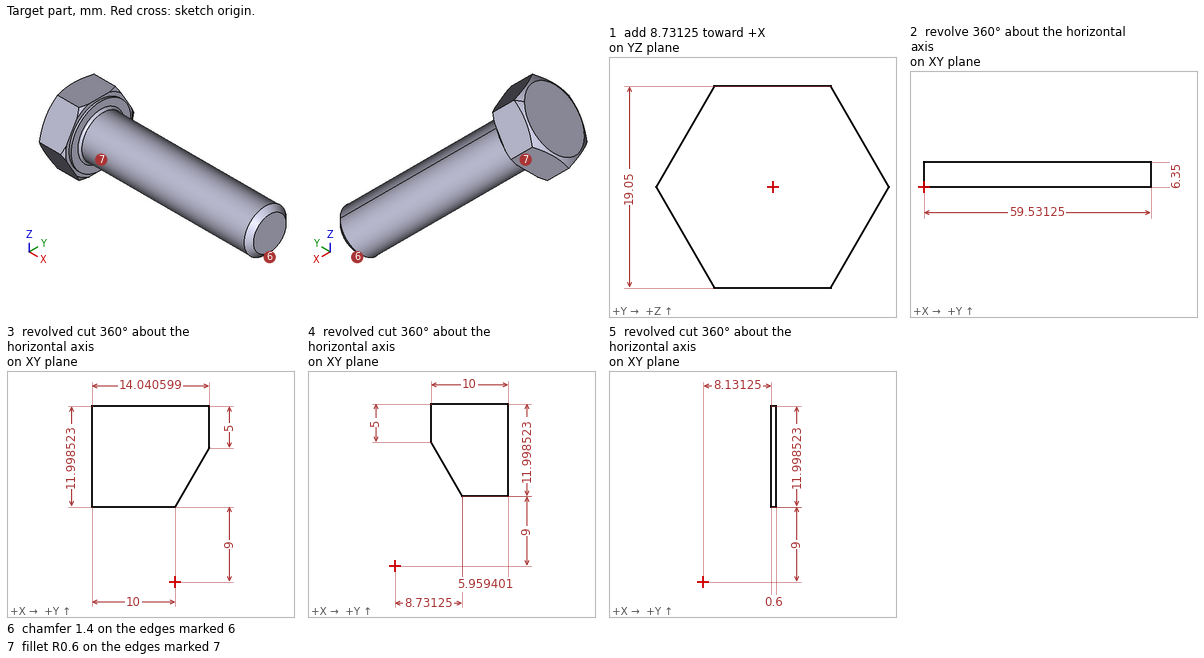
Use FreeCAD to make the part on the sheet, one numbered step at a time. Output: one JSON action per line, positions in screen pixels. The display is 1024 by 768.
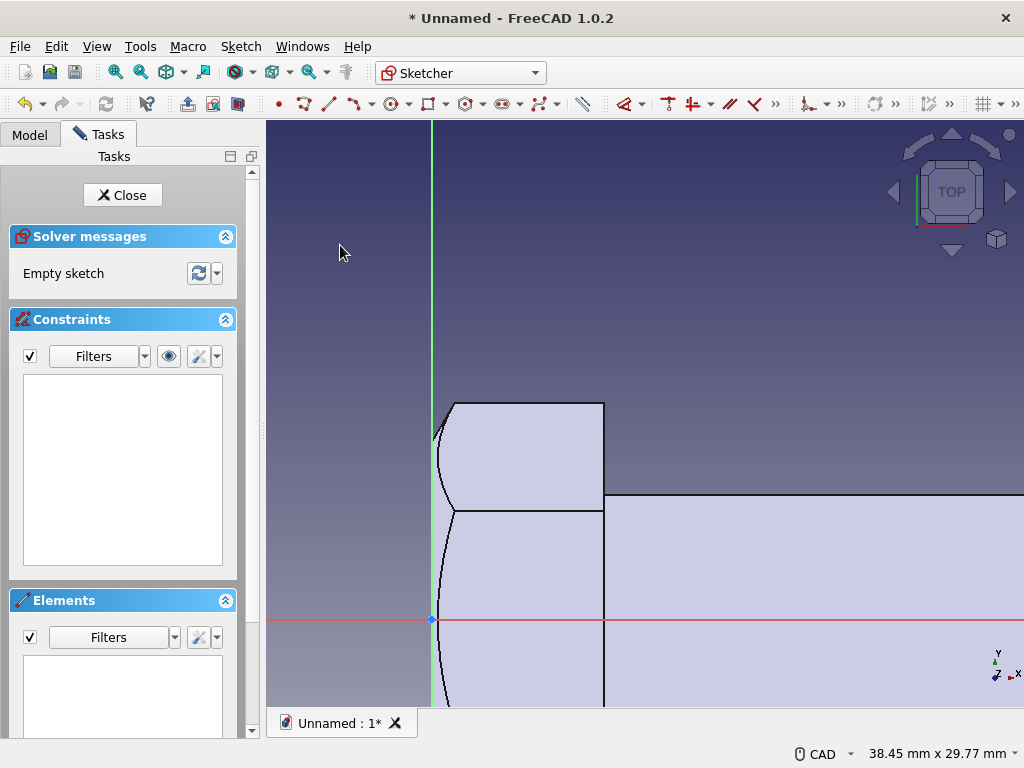
{"action": "left_click", "coordinate": [304, 104]}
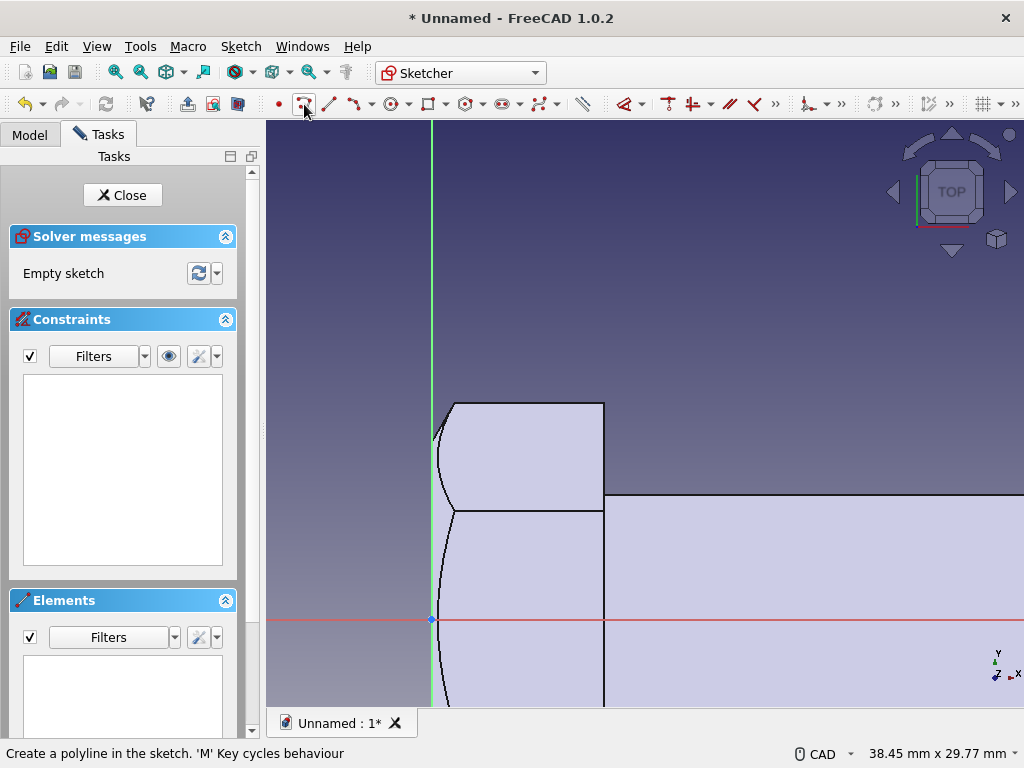
{"action": "left_click", "coordinate": [604, 442]}
{"action": "left_click", "coordinate": [721, 442]}
{"action": "left_click", "coordinate": [721, 206]}
{"action": "left_click", "coordinate": [524, 206]}
{"action": "left_click", "coordinate": [524, 304]}
{"action": "left_click", "coordinate": [604, 443]}
{"action": "key", "text": "Escape"}
{"action": "key", "text": "Escape"}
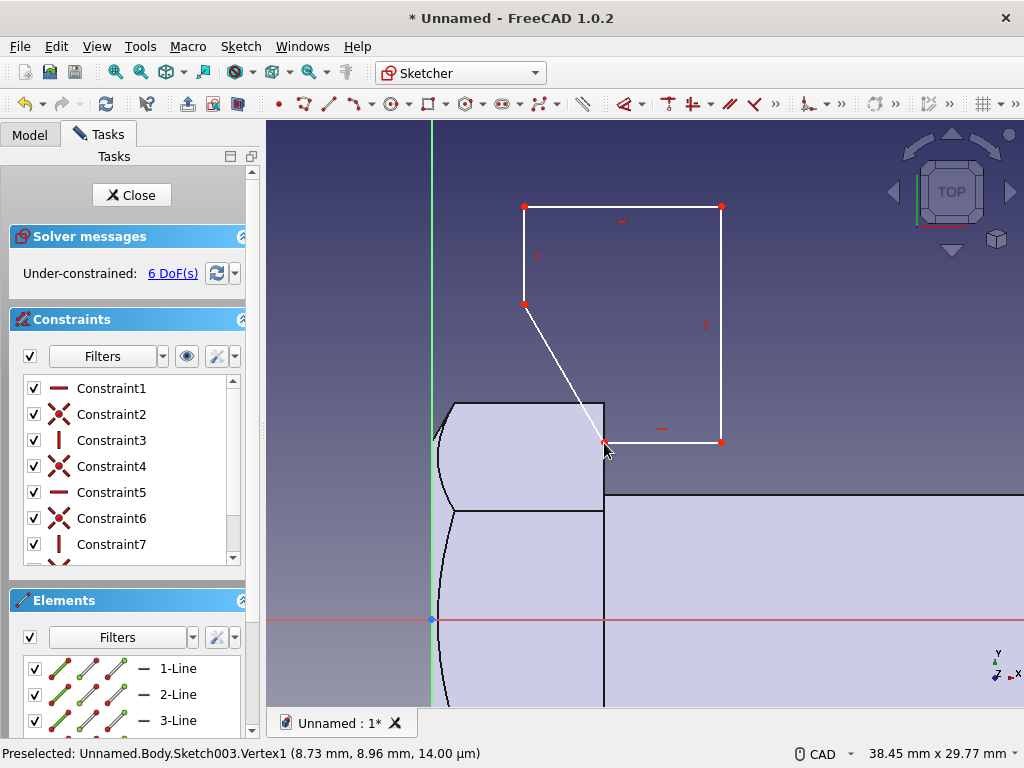
{"action": "left_click", "coordinate": [624, 104]}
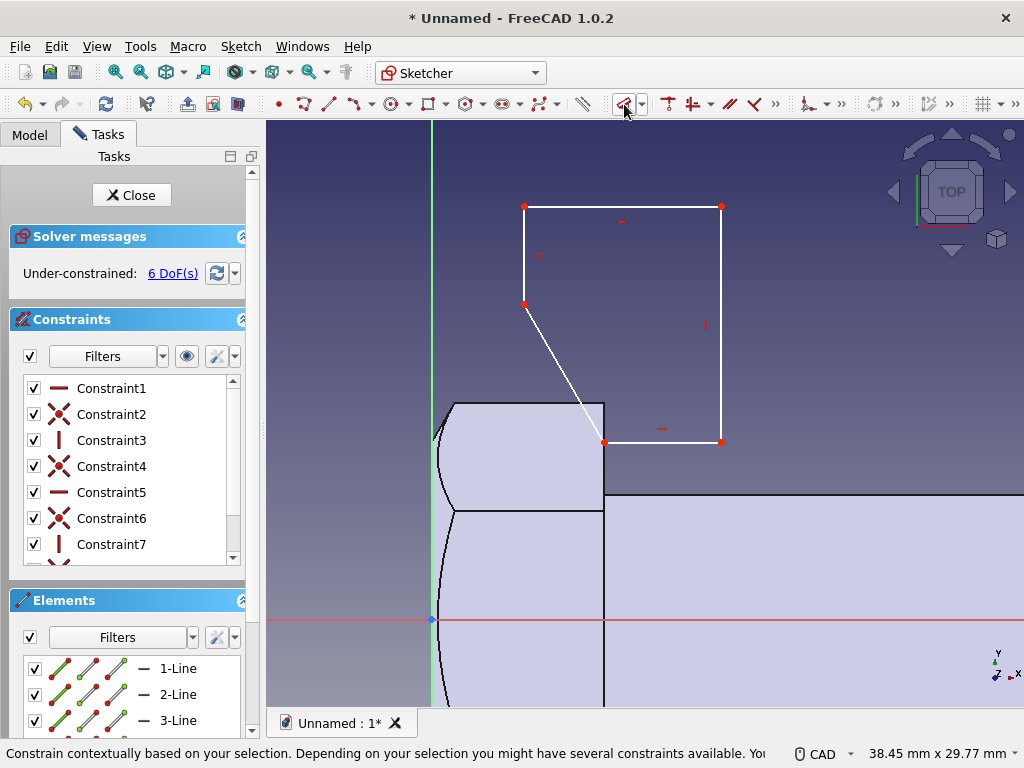
{"action": "left_click", "coordinate": [524, 236]}
{"action": "left_click", "coordinate": [490, 256]}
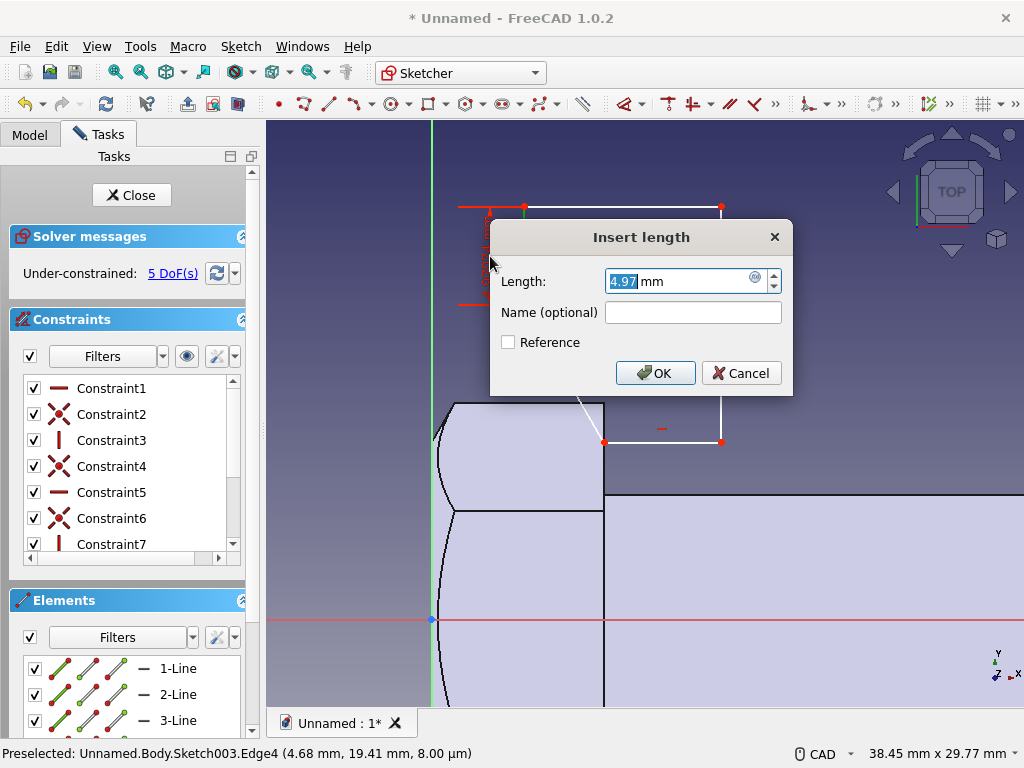
{"action": "type", "text": "5"}
{"action": "key", "text": "Return"}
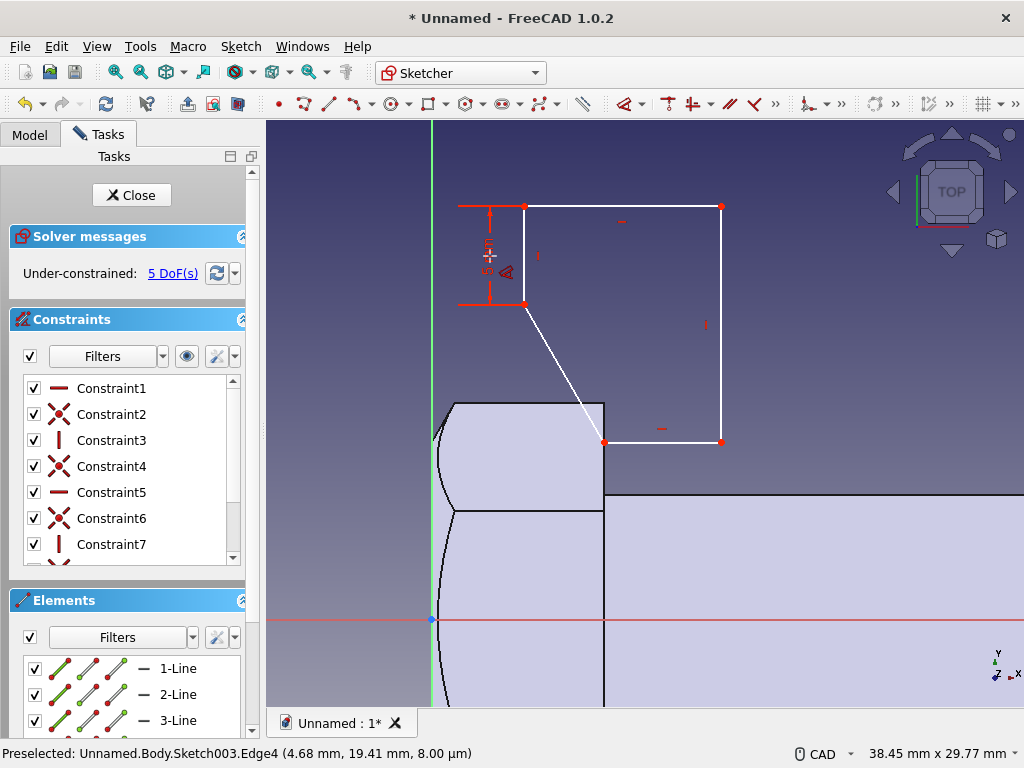
{"action": "left_click", "coordinate": [662, 206]}
{"action": "left_click", "coordinate": [623, 172]}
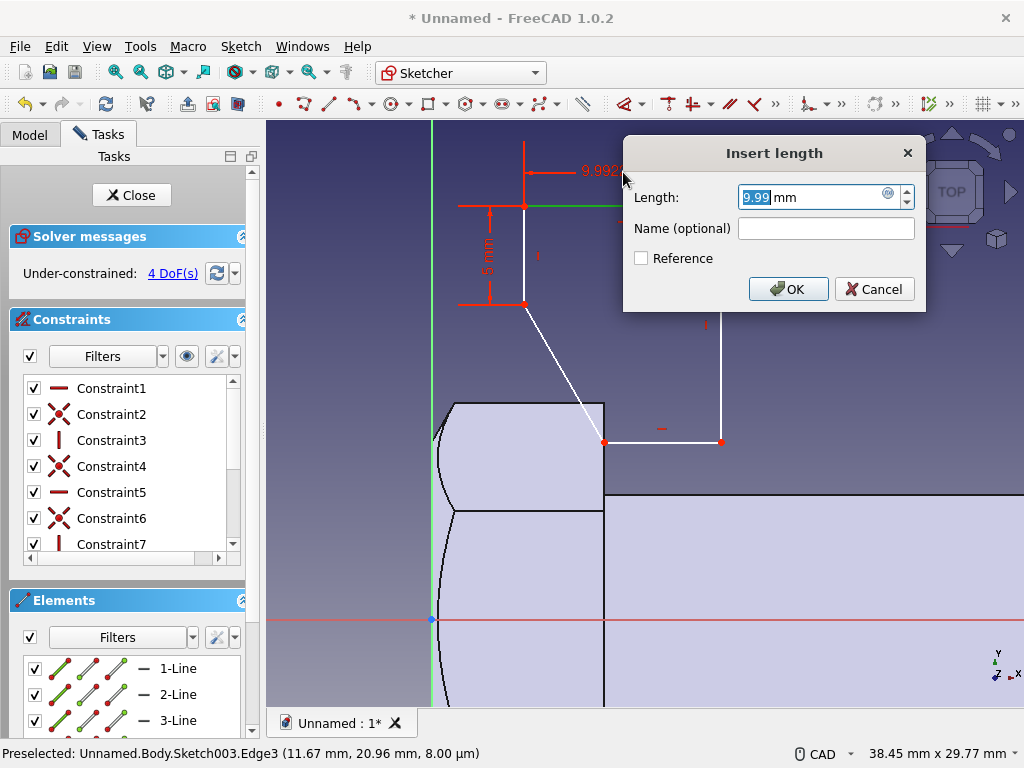
{"action": "type", "text": "10"}
{"action": "key", "text": "Return"}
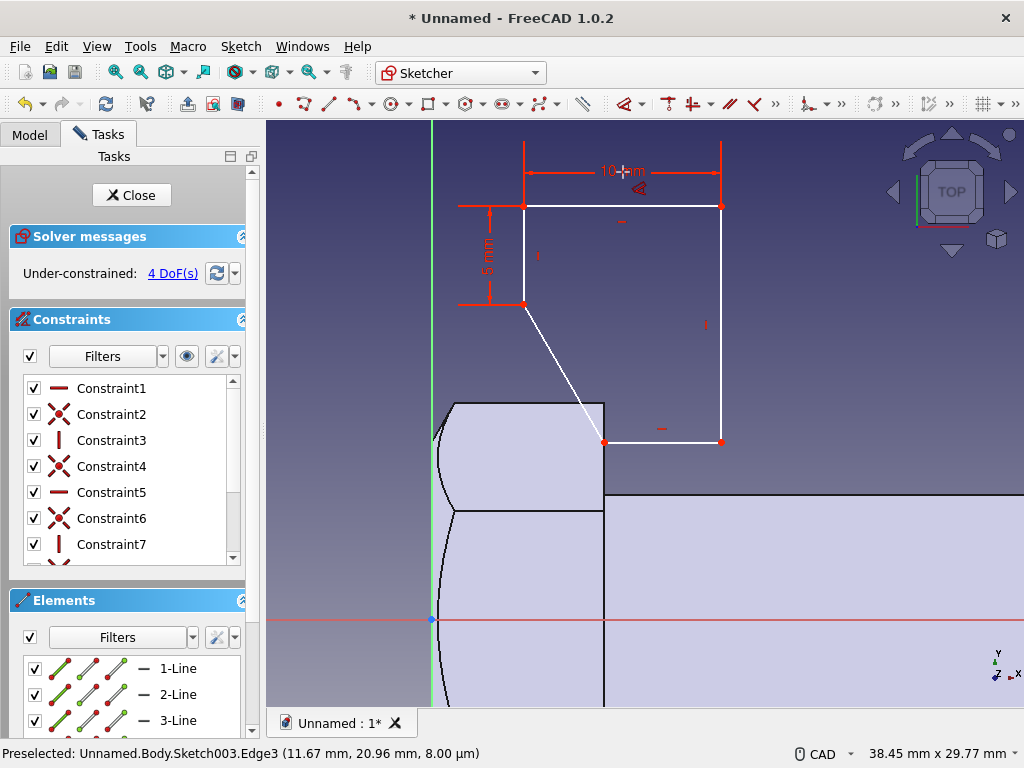
{"action": "left_click", "coordinate": [604, 443]}
{"action": "left_click", "coordinate": [398, 531]}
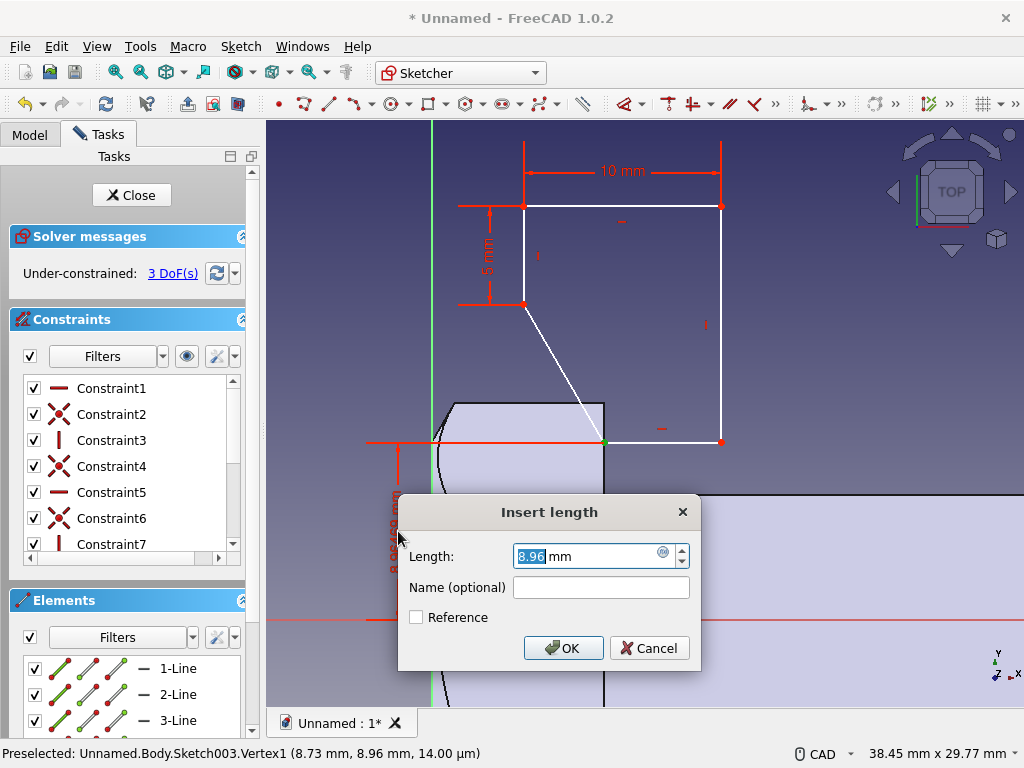
{"action": "type", "text": "9"}
{"action": "key", "text": "Return"}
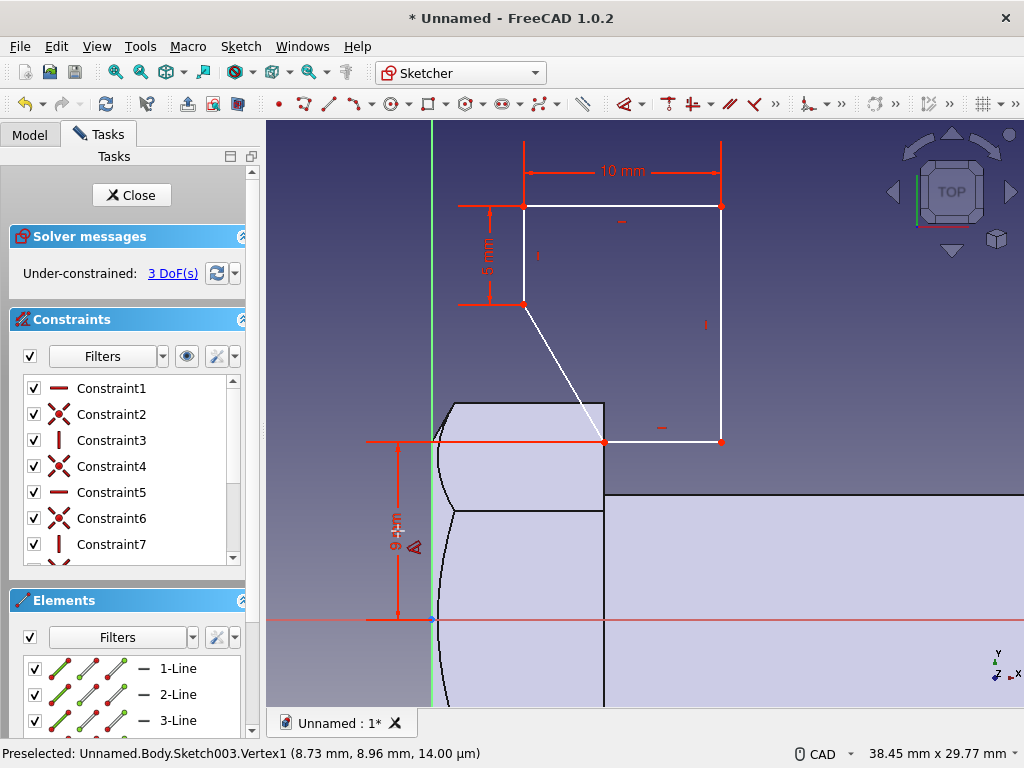
{"action": "left_click", "coordinate": [639, 442]}
{"action": "left_click", "coordinate": [662, 476]}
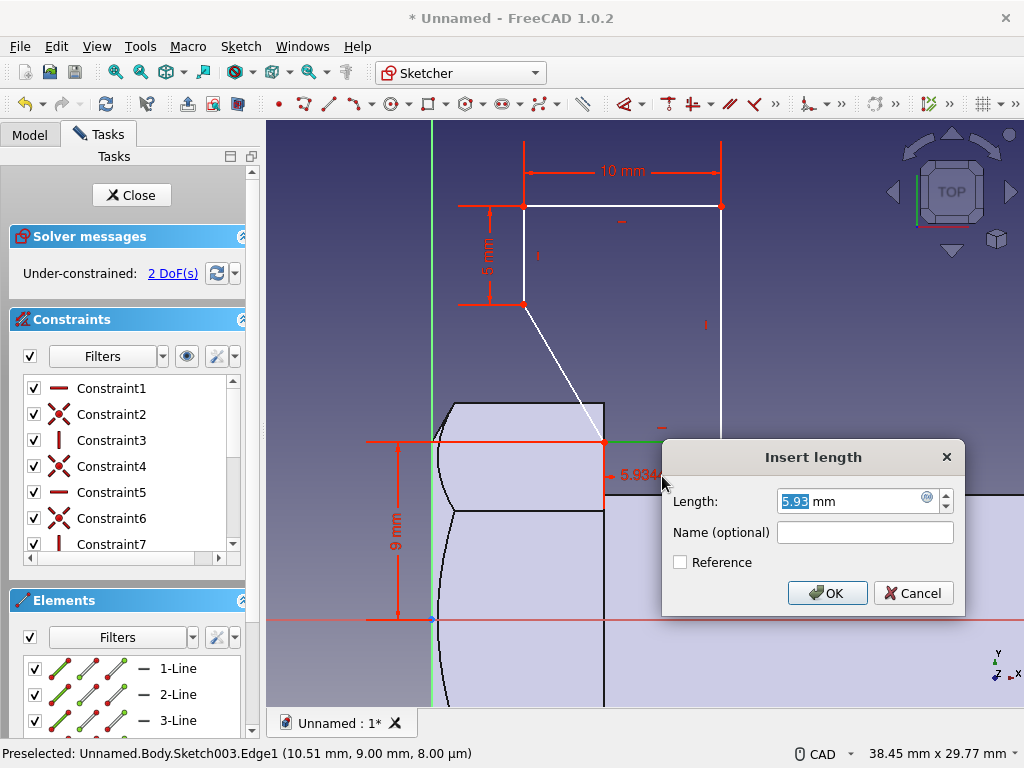
{"action": "type", "text": "5.959401"}
{"action": "key", "text": "Return"}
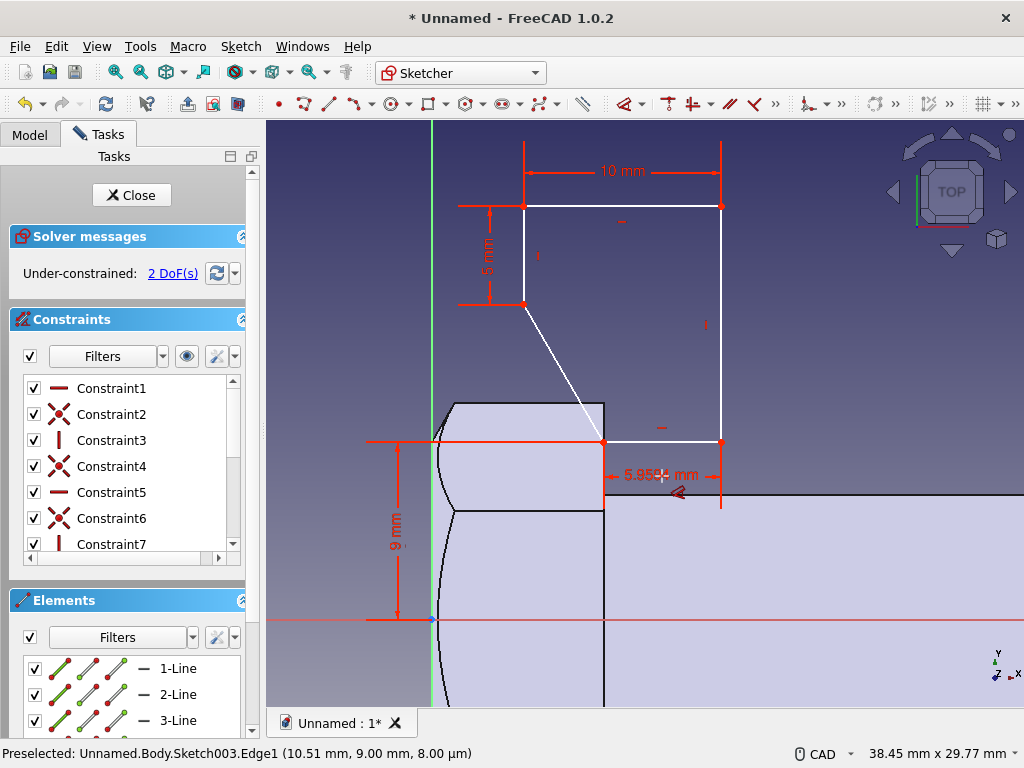
{"action": "left_click", "coordinate": [604, 442]}
{"action": "left_click", "coordinate": [518, 654]}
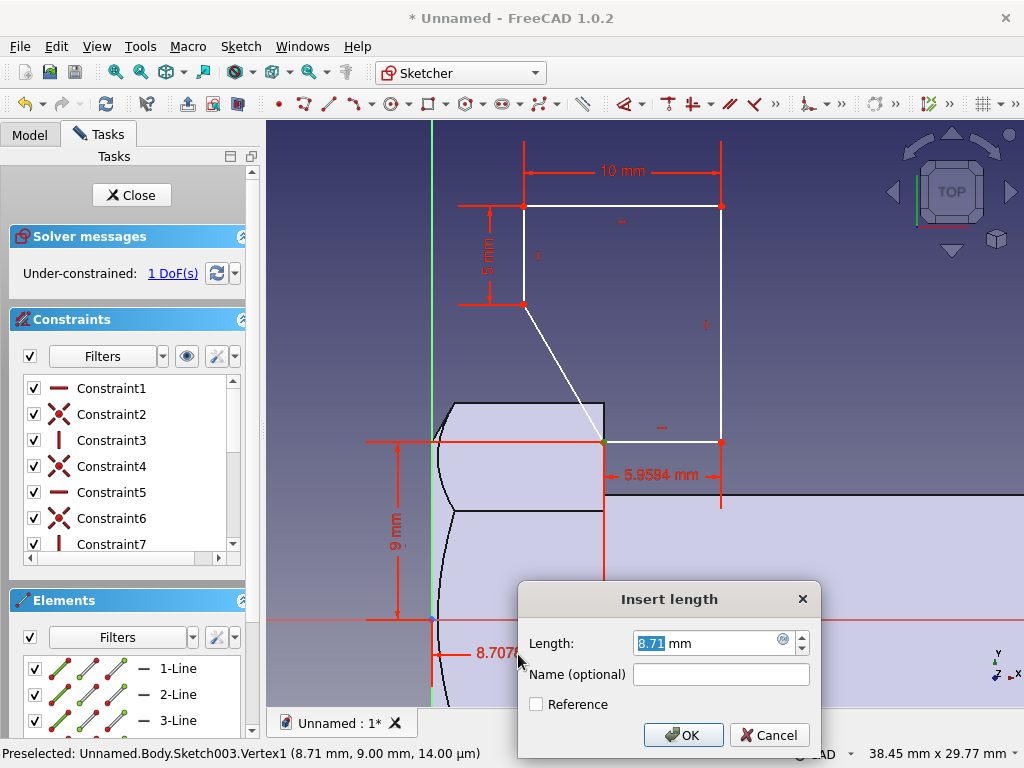
{"action": "type", "text": "8.73125"}
{"action": "key", "text": "Return"}